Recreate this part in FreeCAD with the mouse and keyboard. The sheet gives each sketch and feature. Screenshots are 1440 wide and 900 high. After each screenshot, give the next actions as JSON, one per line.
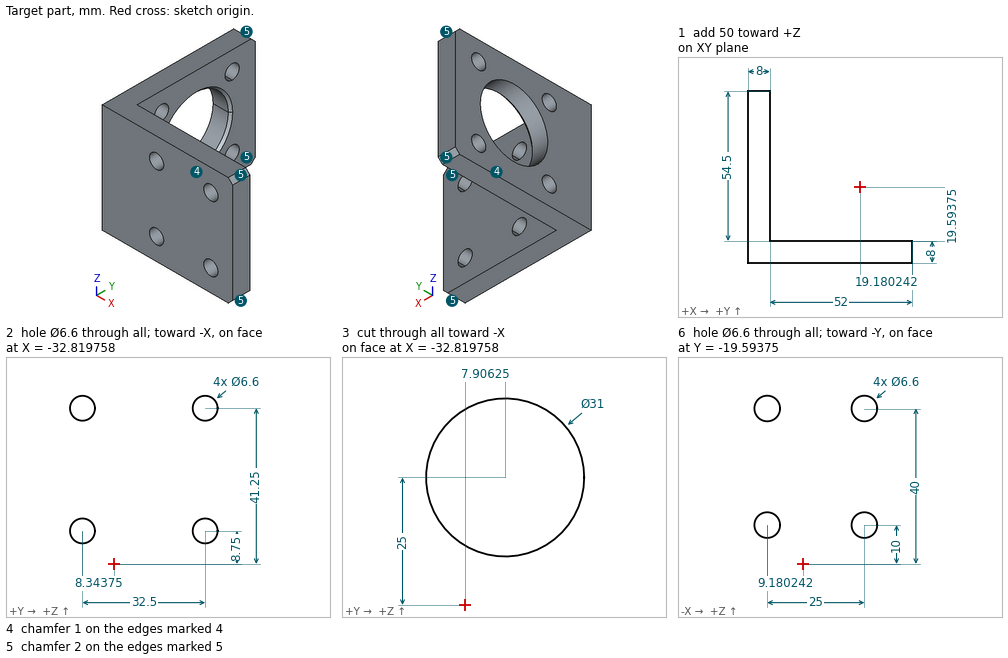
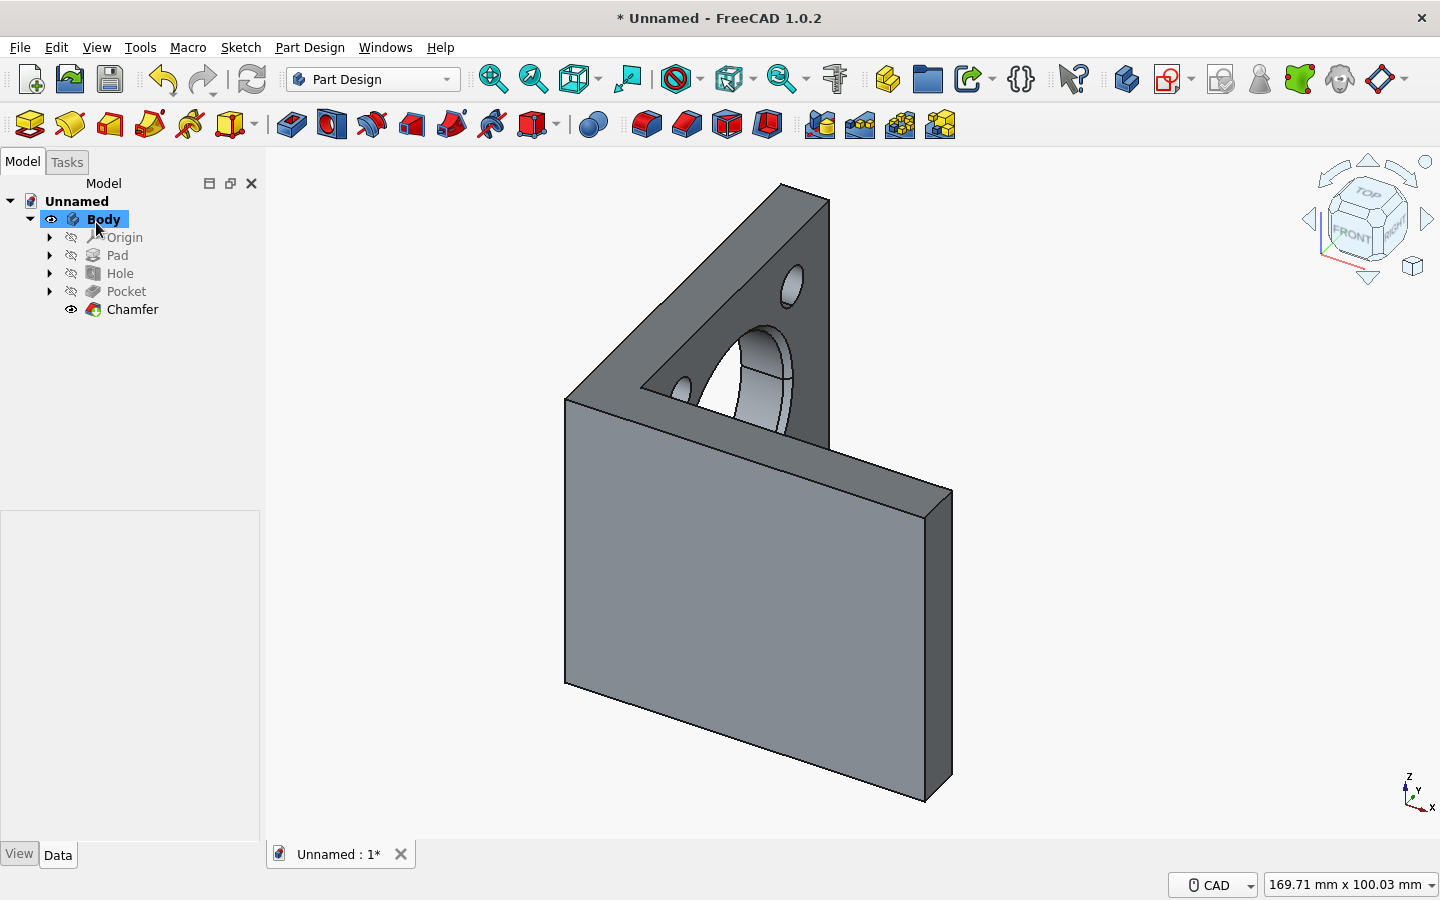
{"action": "left_click", "coordinate": [938, 503]}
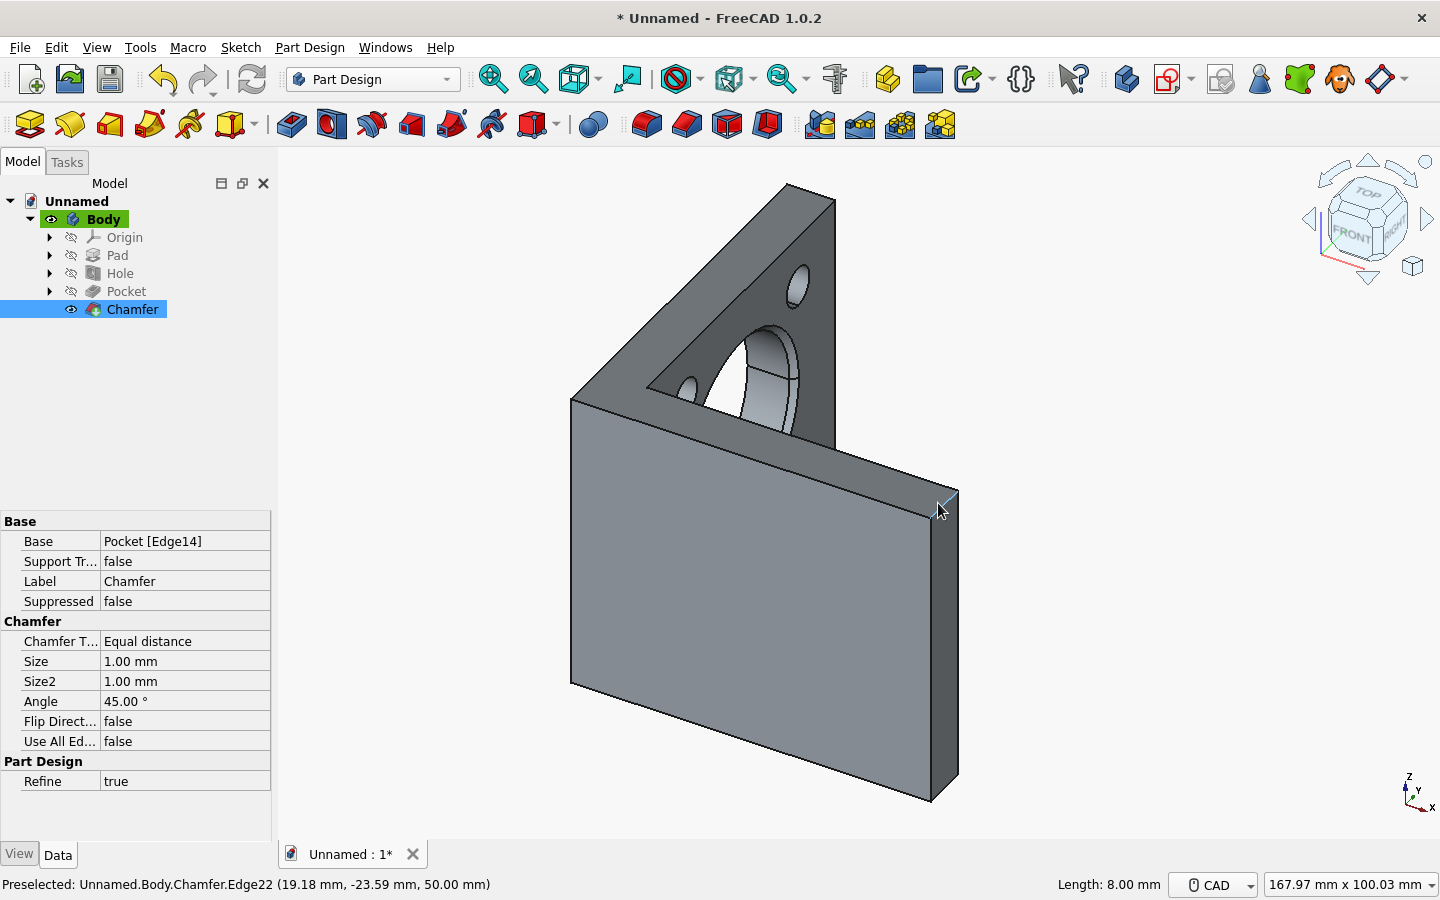
{"action": "key", "text": "0"}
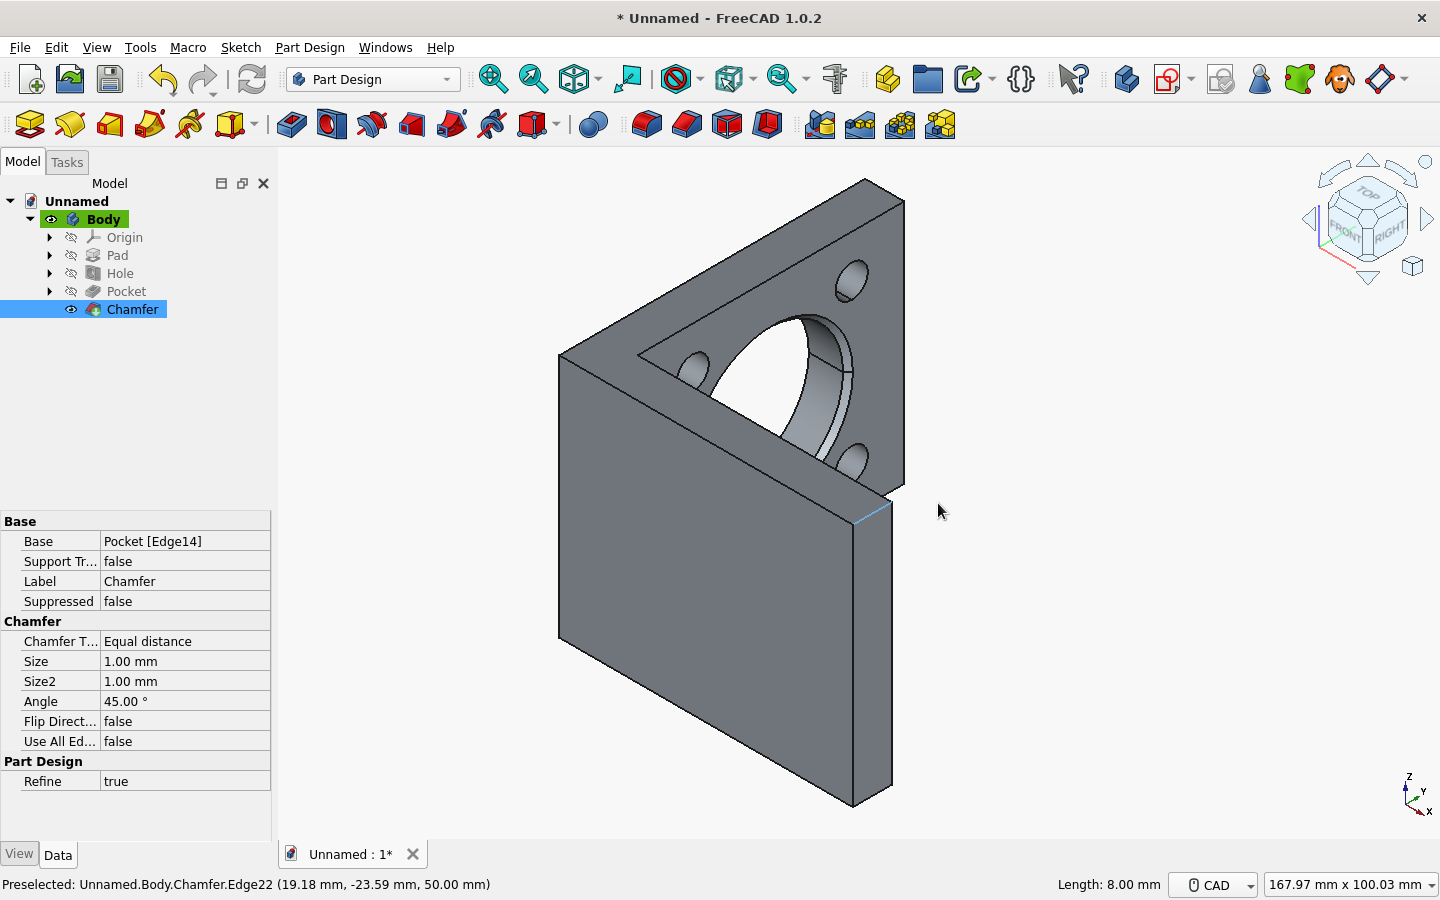
{"action": "key", "text": "2"}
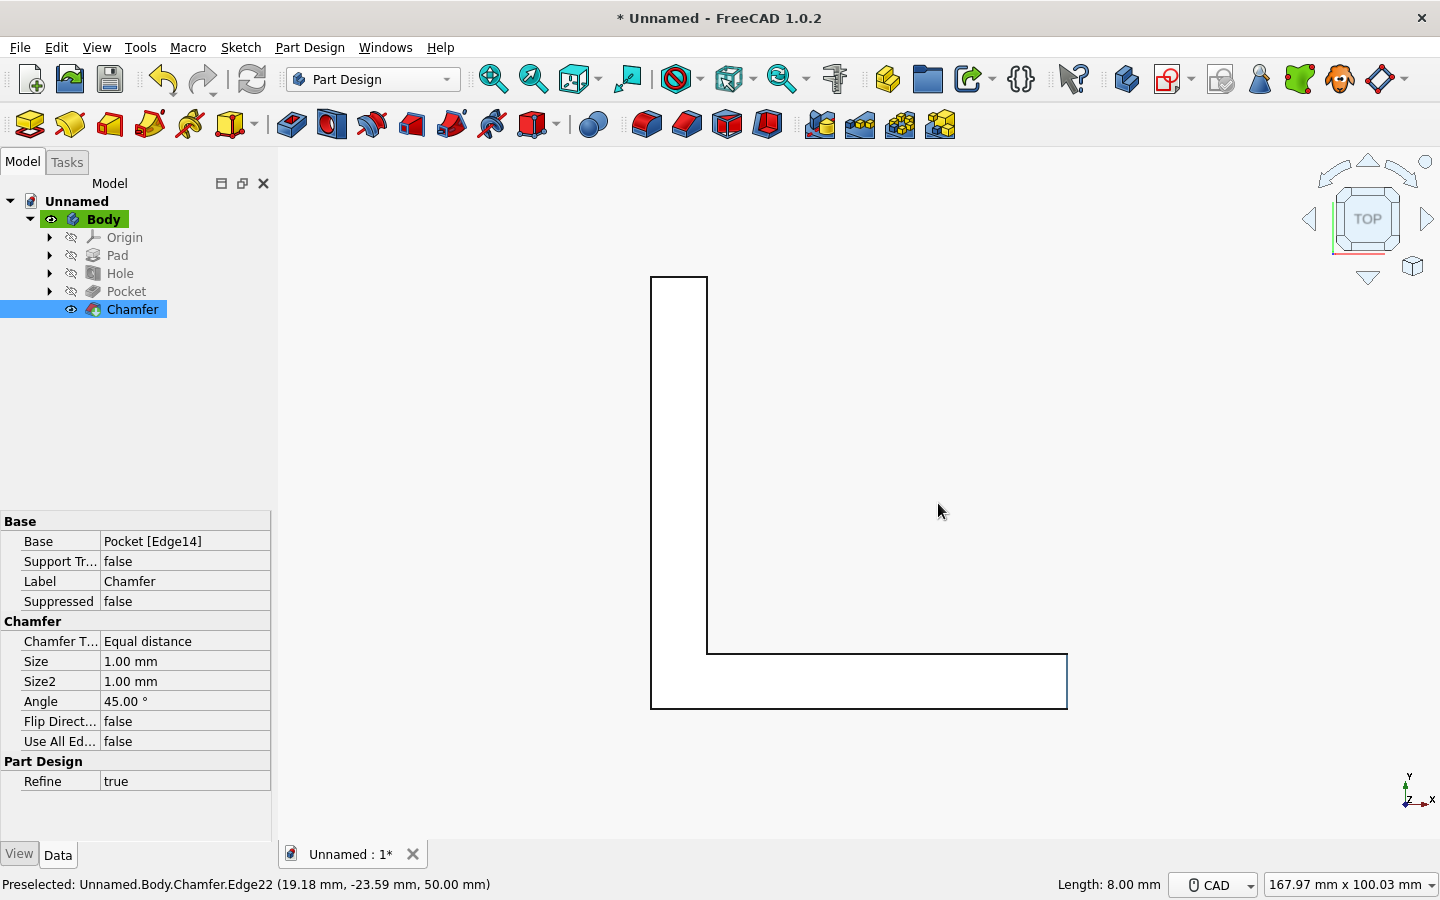
{"action": "left_click", "coordinate": [679, 276], "text": "ctrl"}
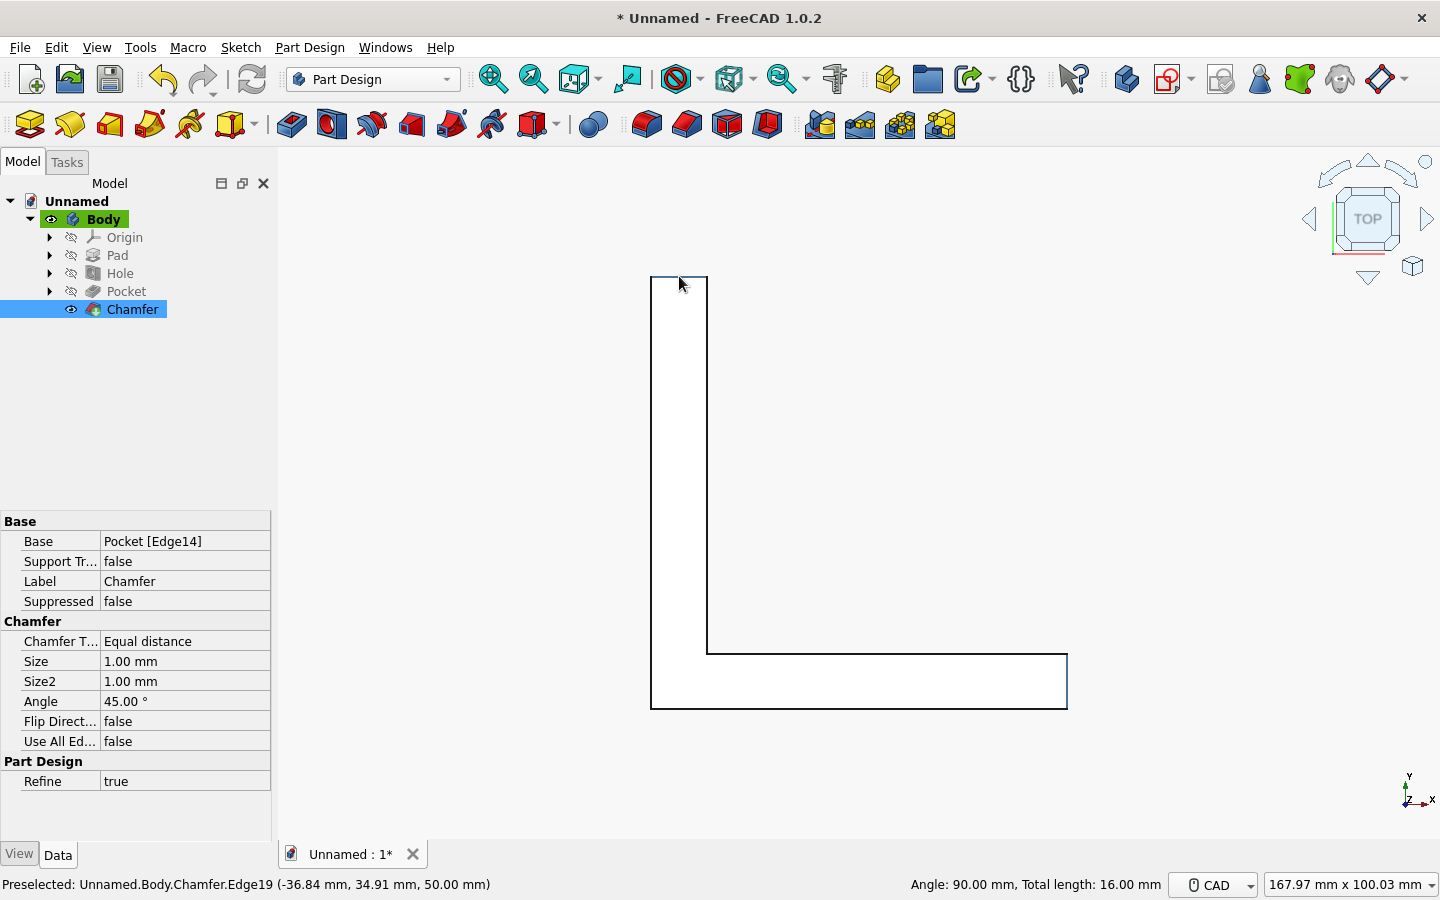
{"action": "key", "text": "1"}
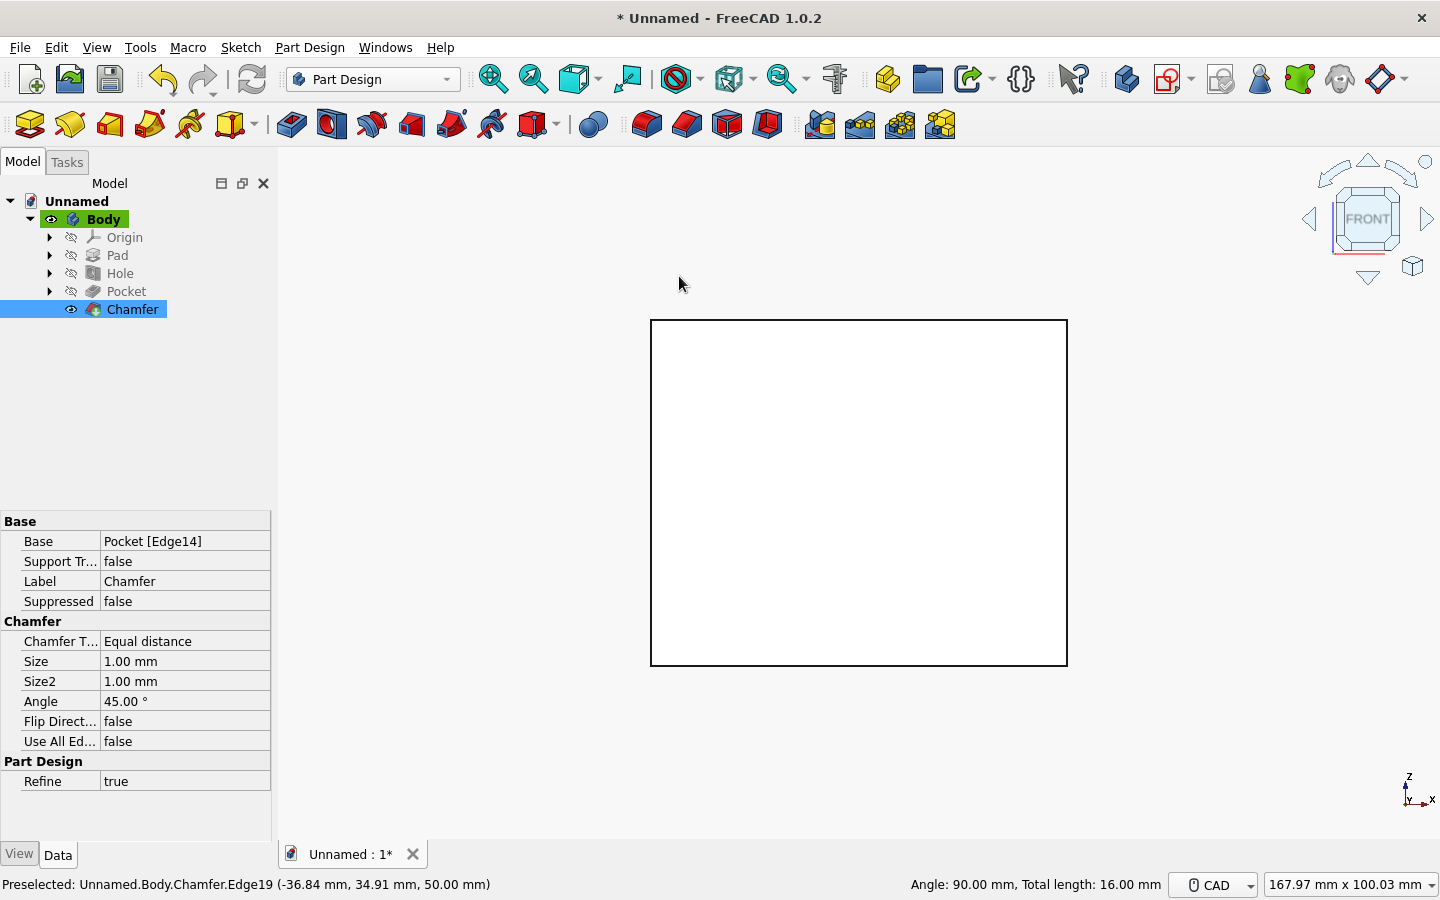
{"action": "key", "text": "3"}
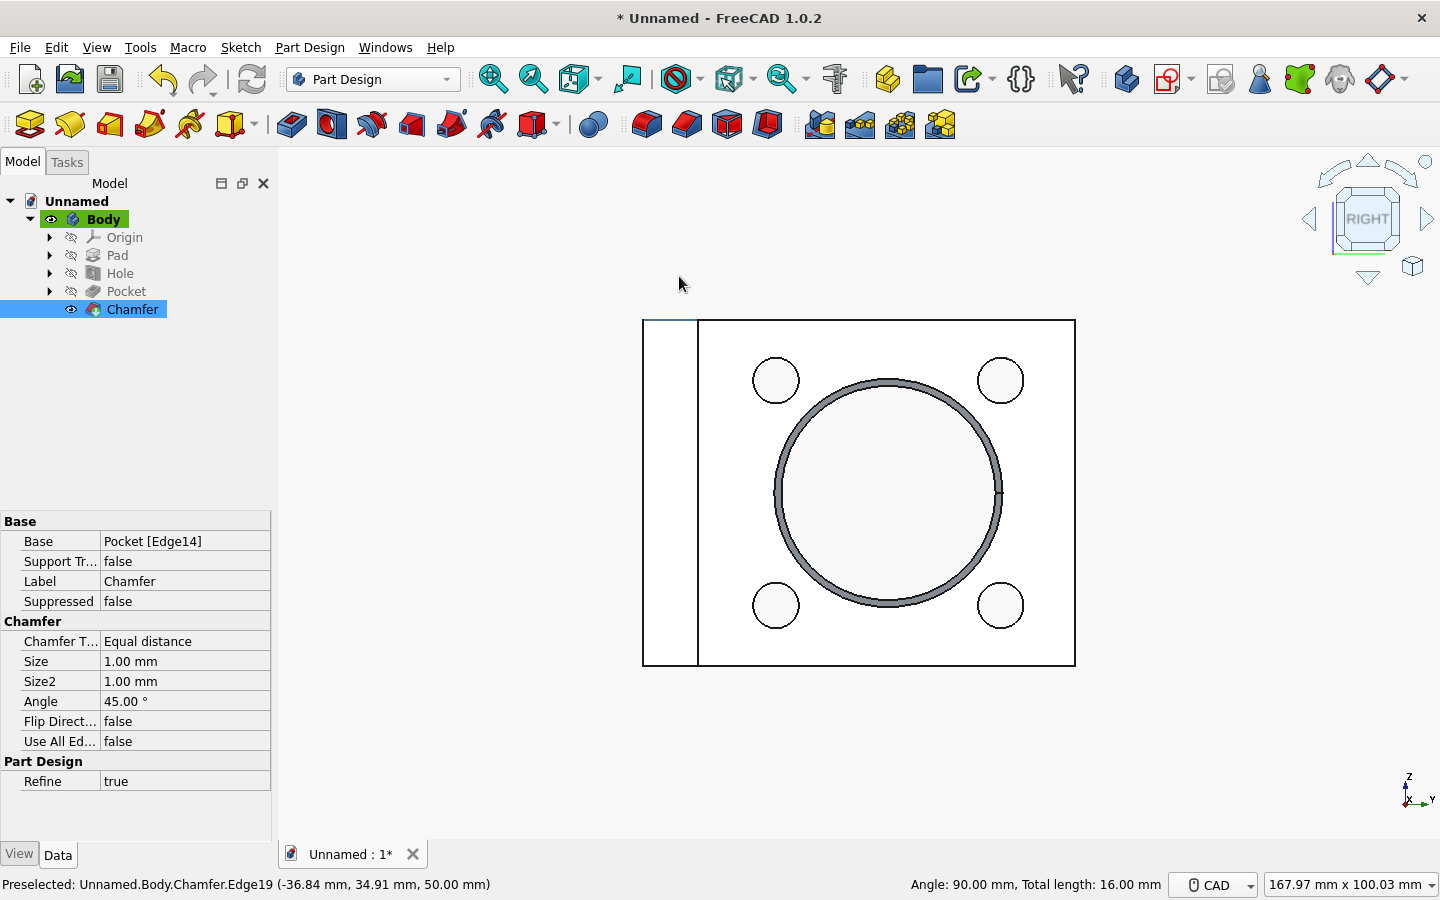
{"action": "left_click", "coordinate": [670, 665], "text": "ctrl"}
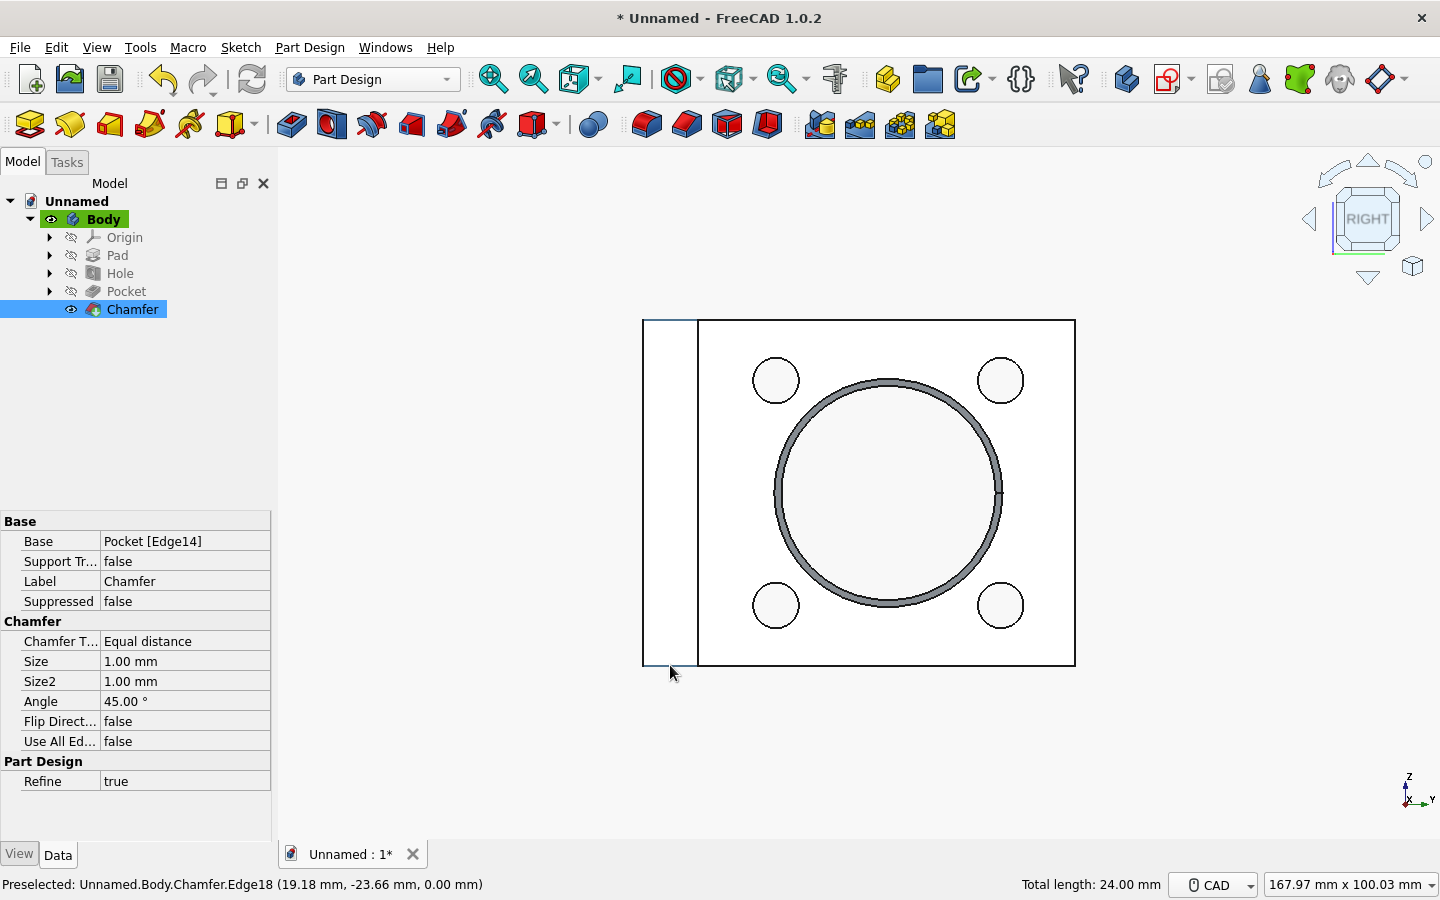
{"action": "key", "text": "5"}